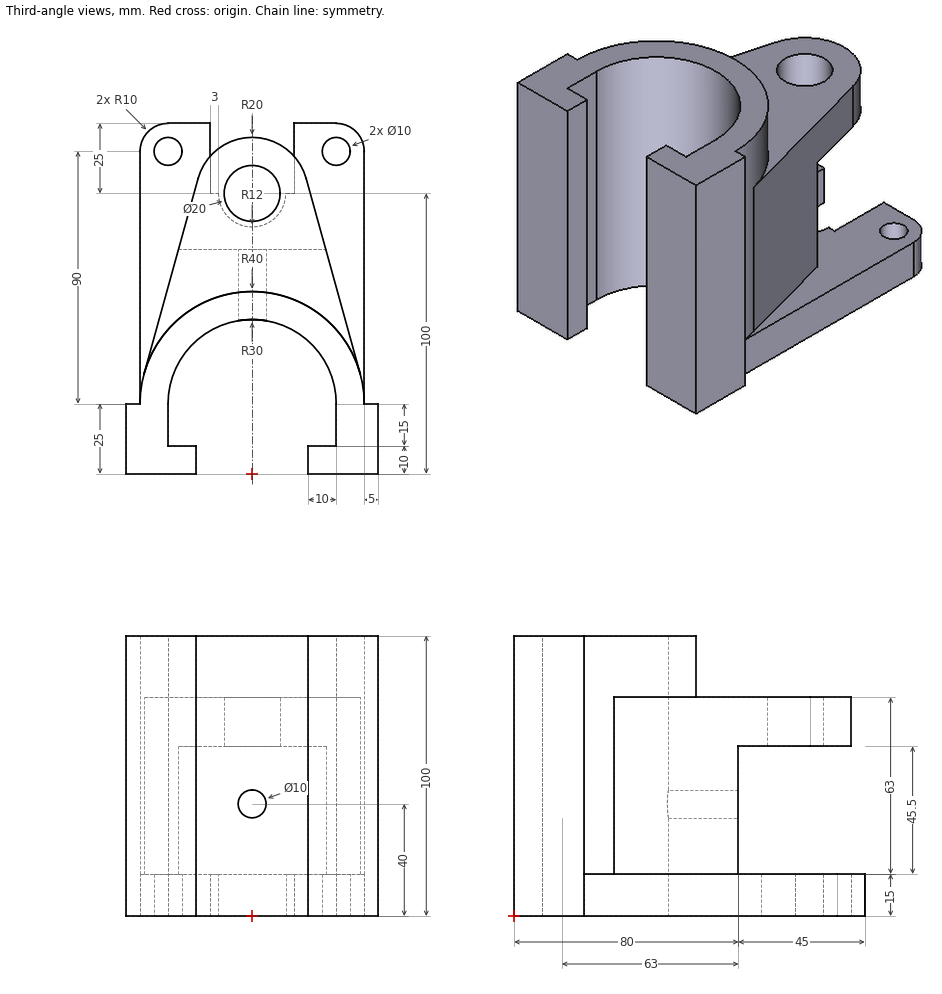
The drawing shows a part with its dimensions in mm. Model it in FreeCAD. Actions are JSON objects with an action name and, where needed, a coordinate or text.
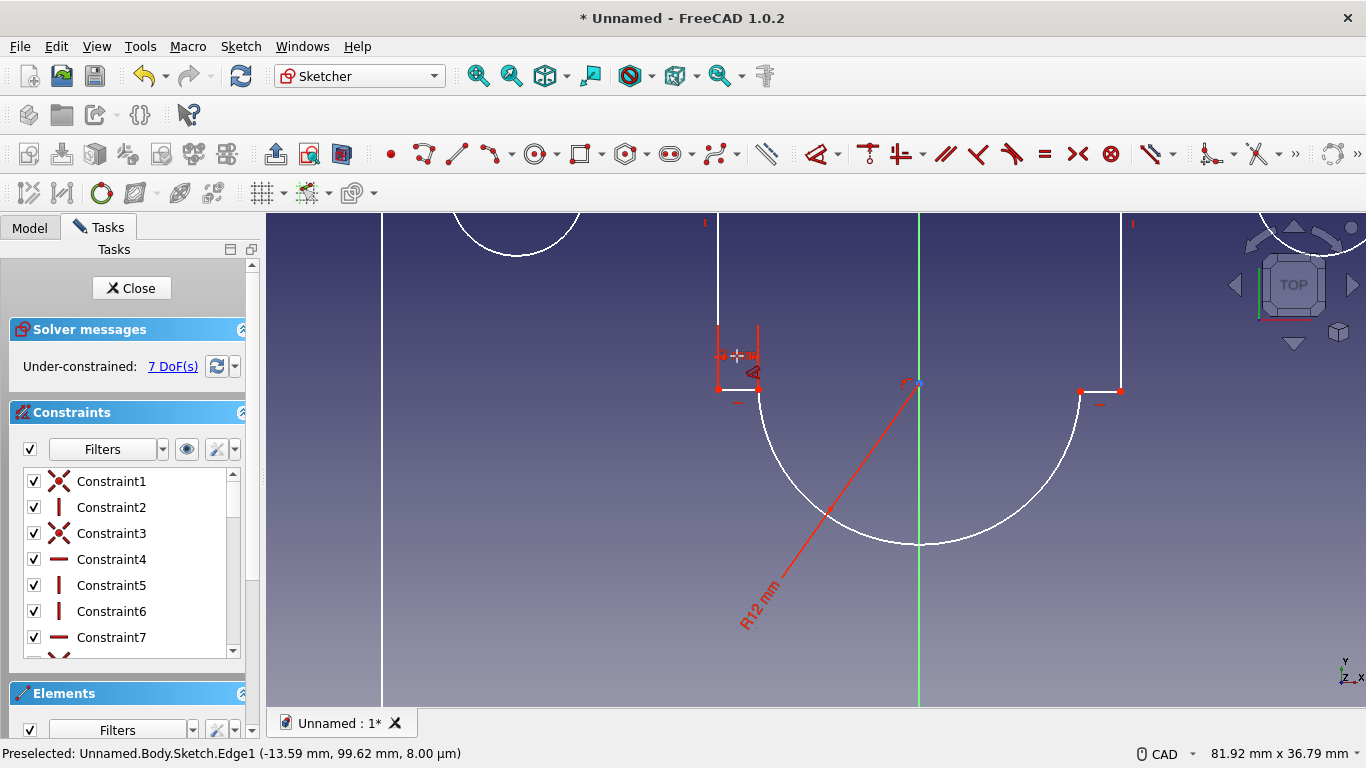
{"action": "scroll", "coordinate": [704, 352], "scroll_direction": "down", "scroll_amount": 8}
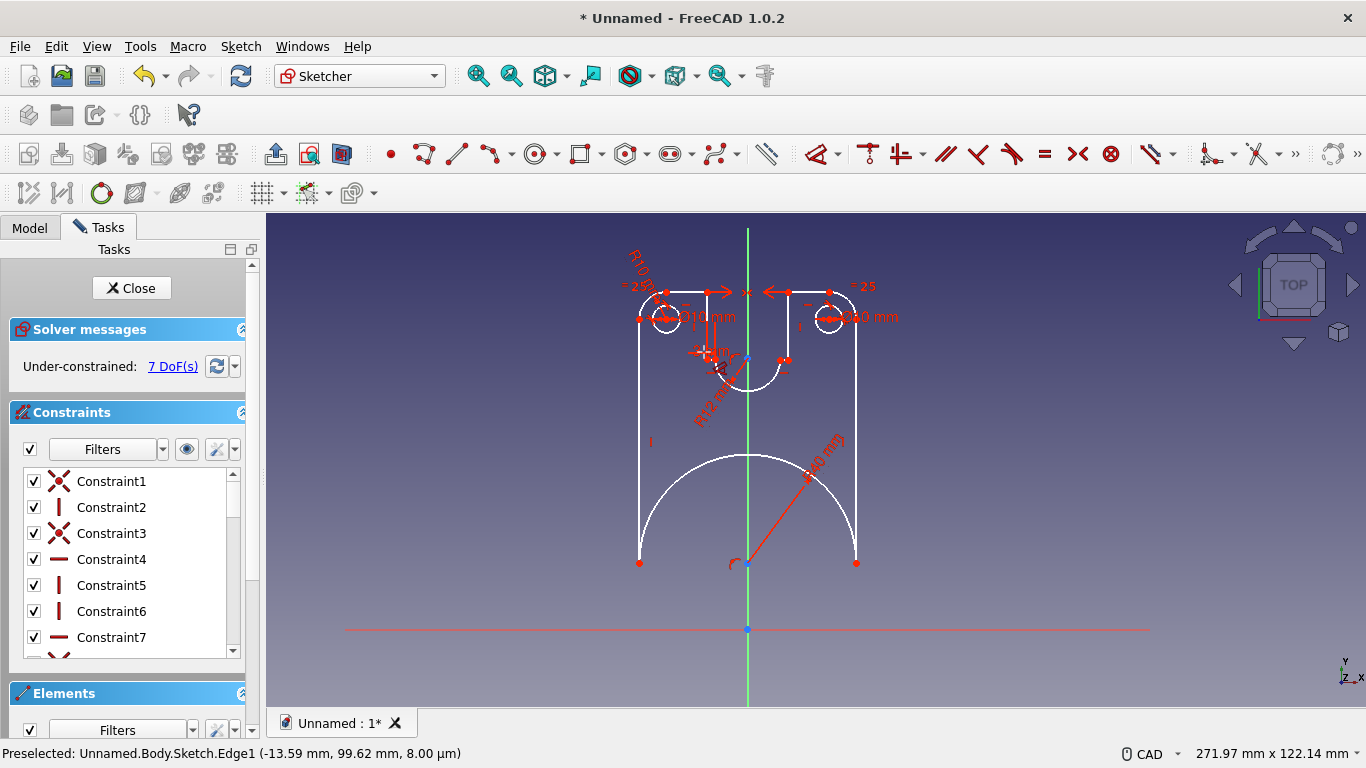
{"action": "left_click", "coordinate": [707, 340]}
{"action": "left_click", "coordinate": [765, 326]}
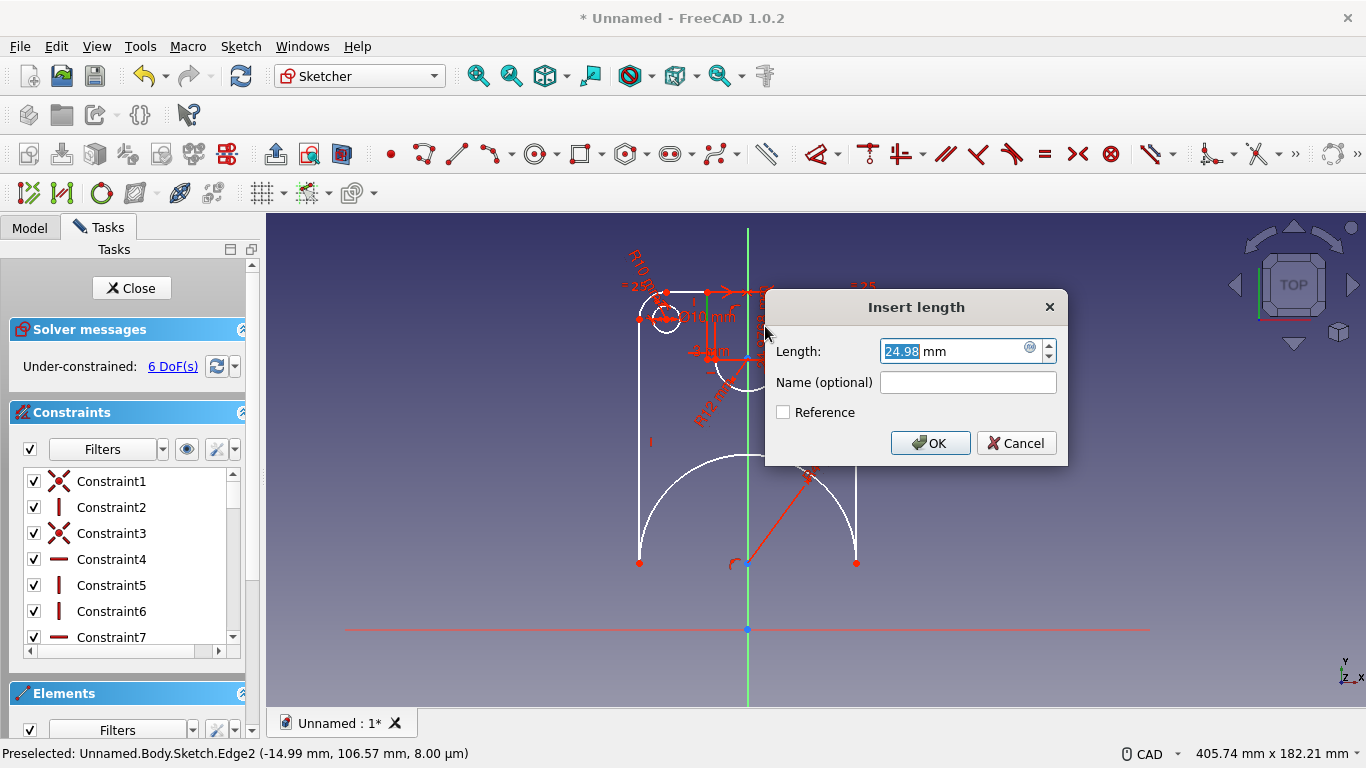
{"action": "type", "text": "25"}
{"action": "key", "text": "Return"}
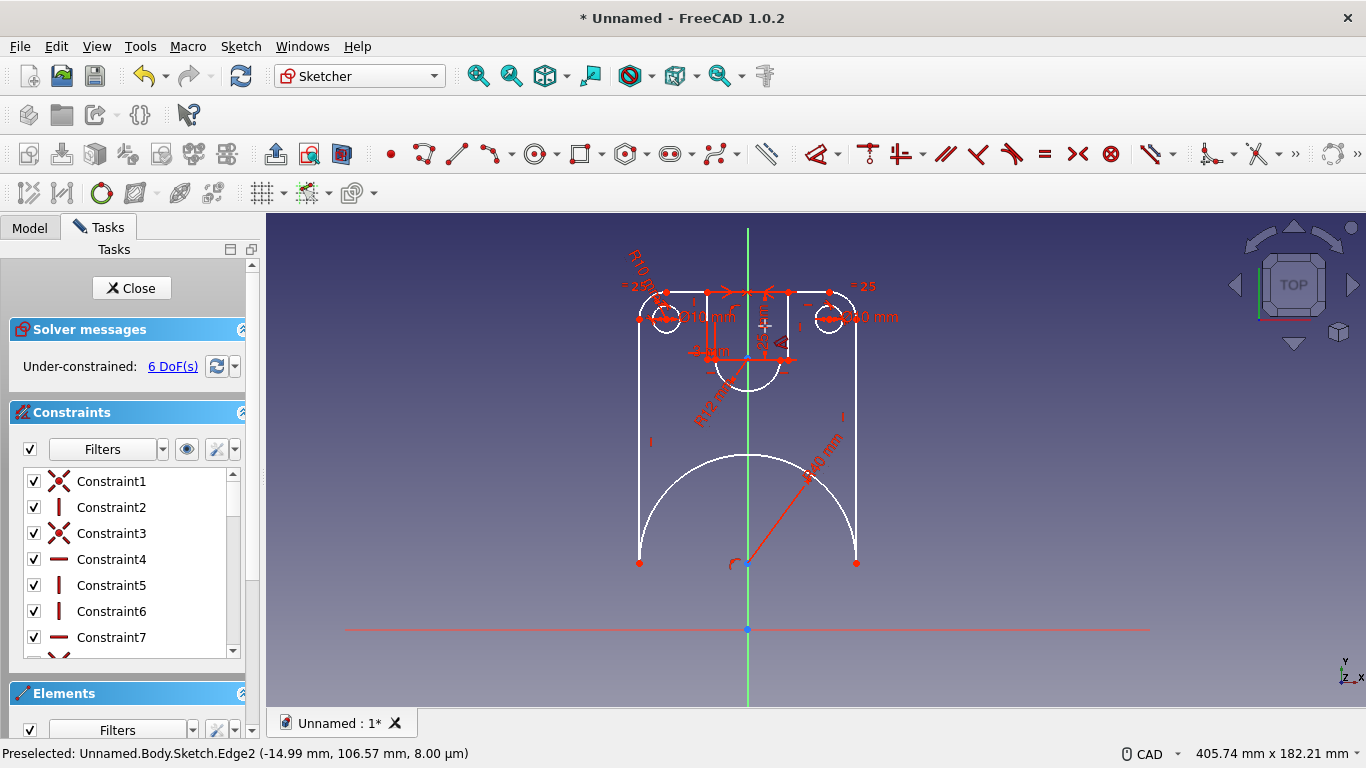
{"action": "left_click", "coordinate": [639, 392]}
{"action": "left_click", "coordinate": [605, 441]}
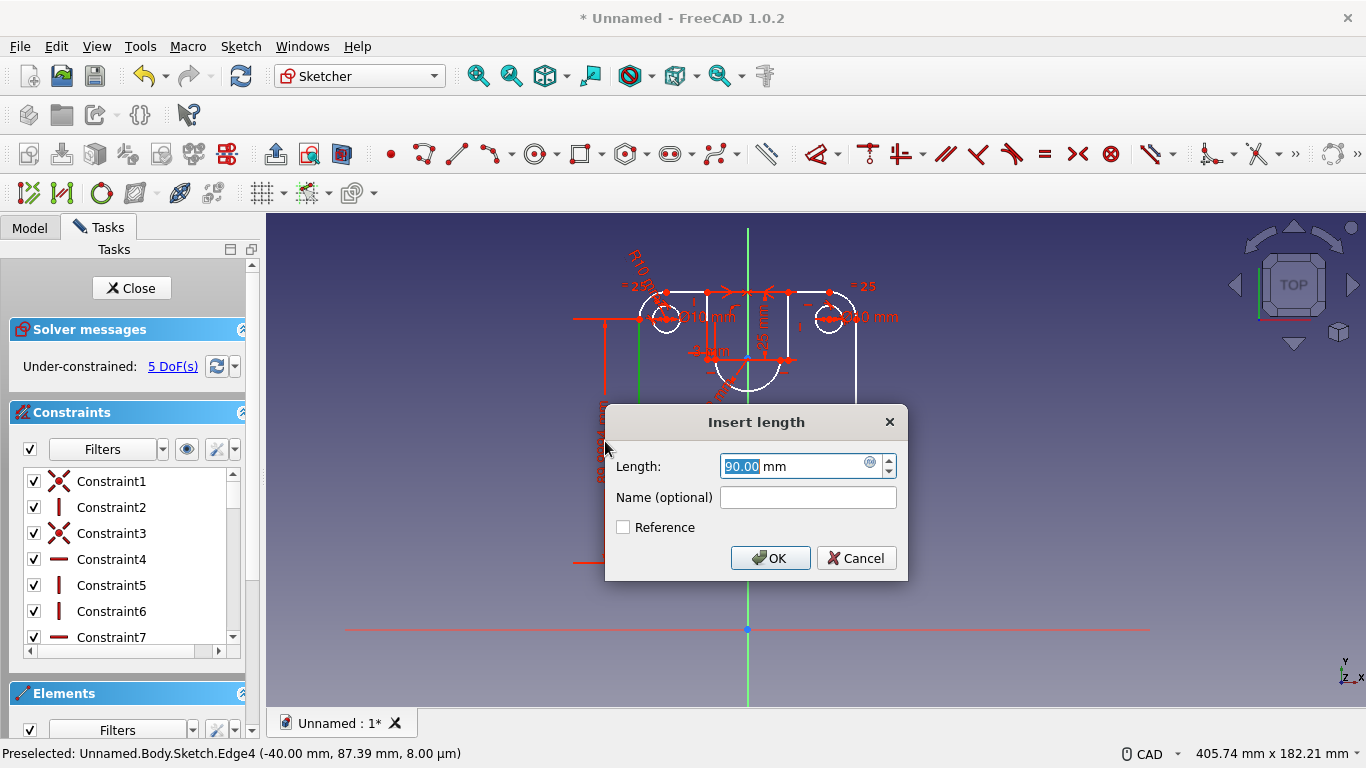
{"action": "type", "text": "90"}
{"action": "key", "text": "Return"}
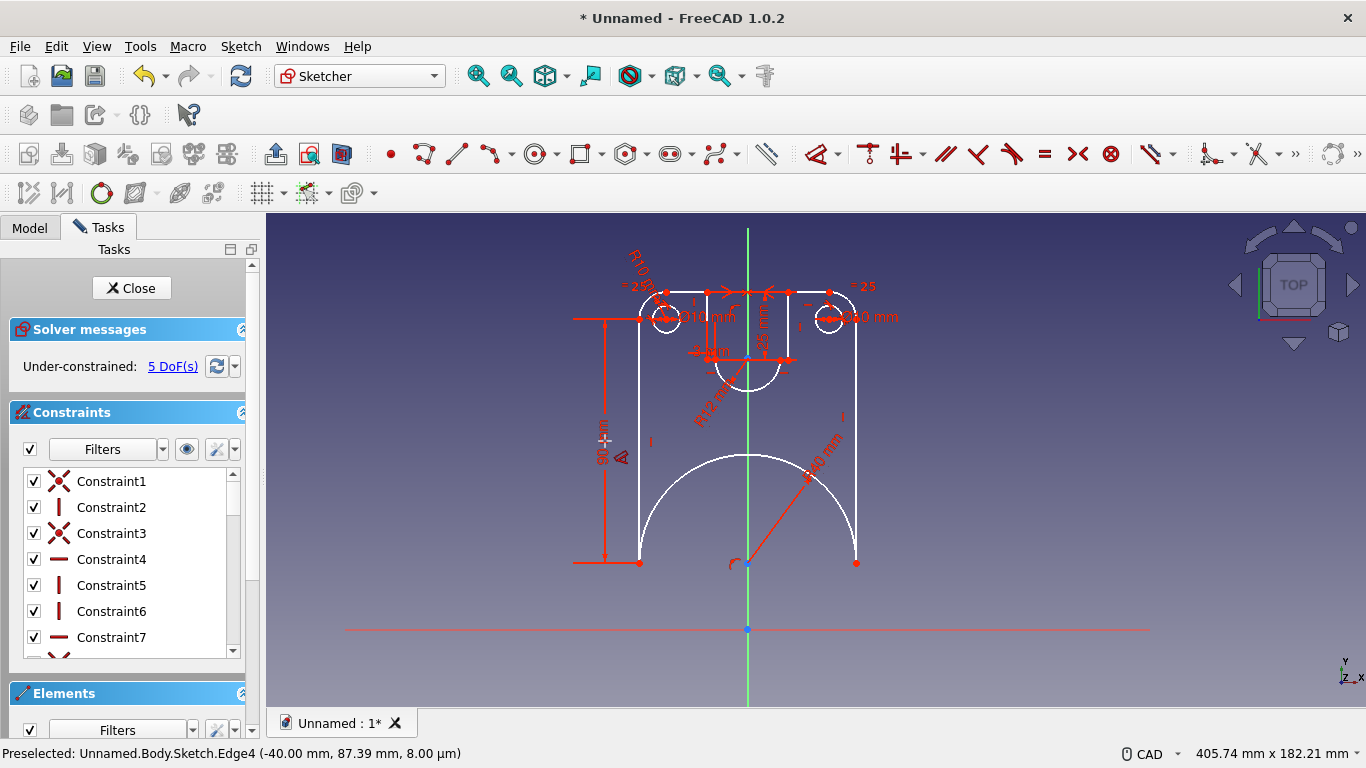
{"action": "left_click", "coordinate": [856, 490]}
{"action": "left_click", "coordinate": [890, 385]}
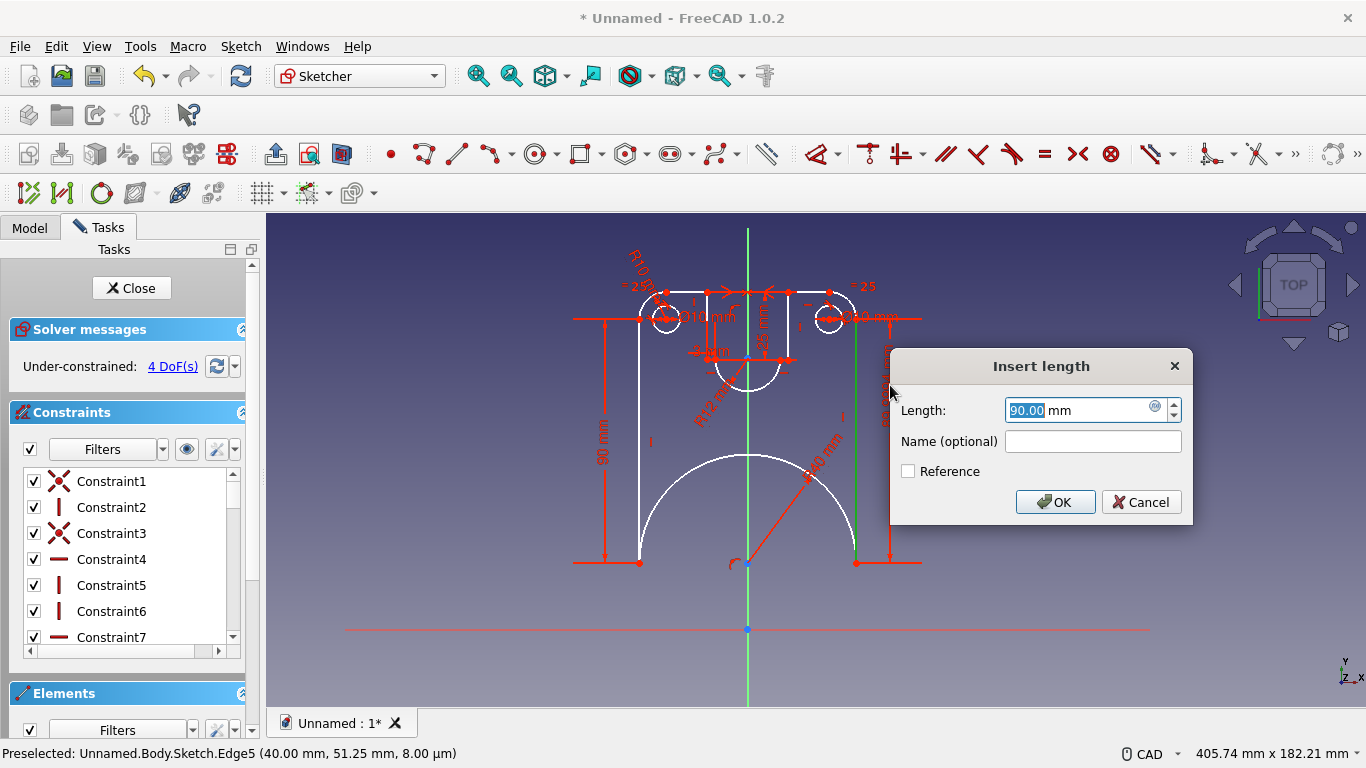
{"action": "type", "text": "90"}
{"action": "key", "text": "Return"}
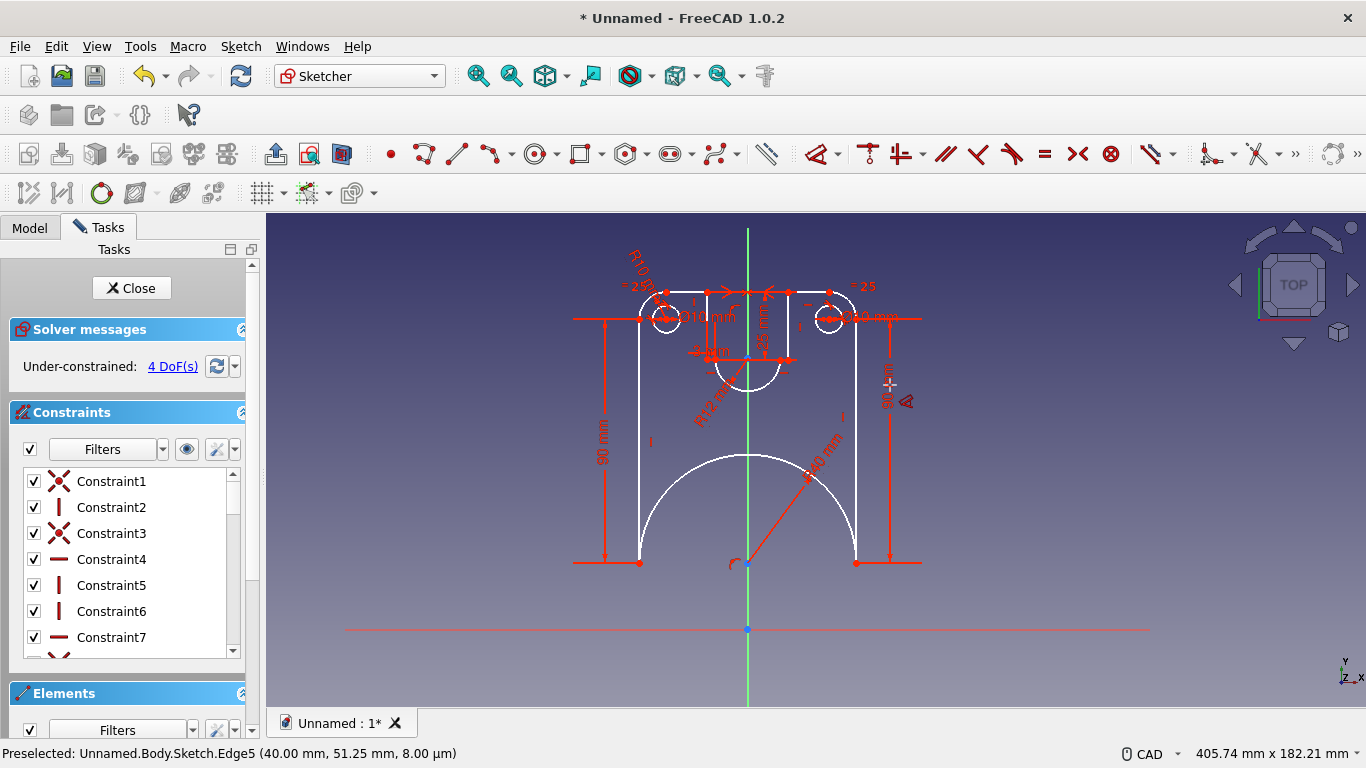
{"action": "left_click", "coordinate": [788, 313]}
{"action": "left_click", "coordinate": [822, 350]}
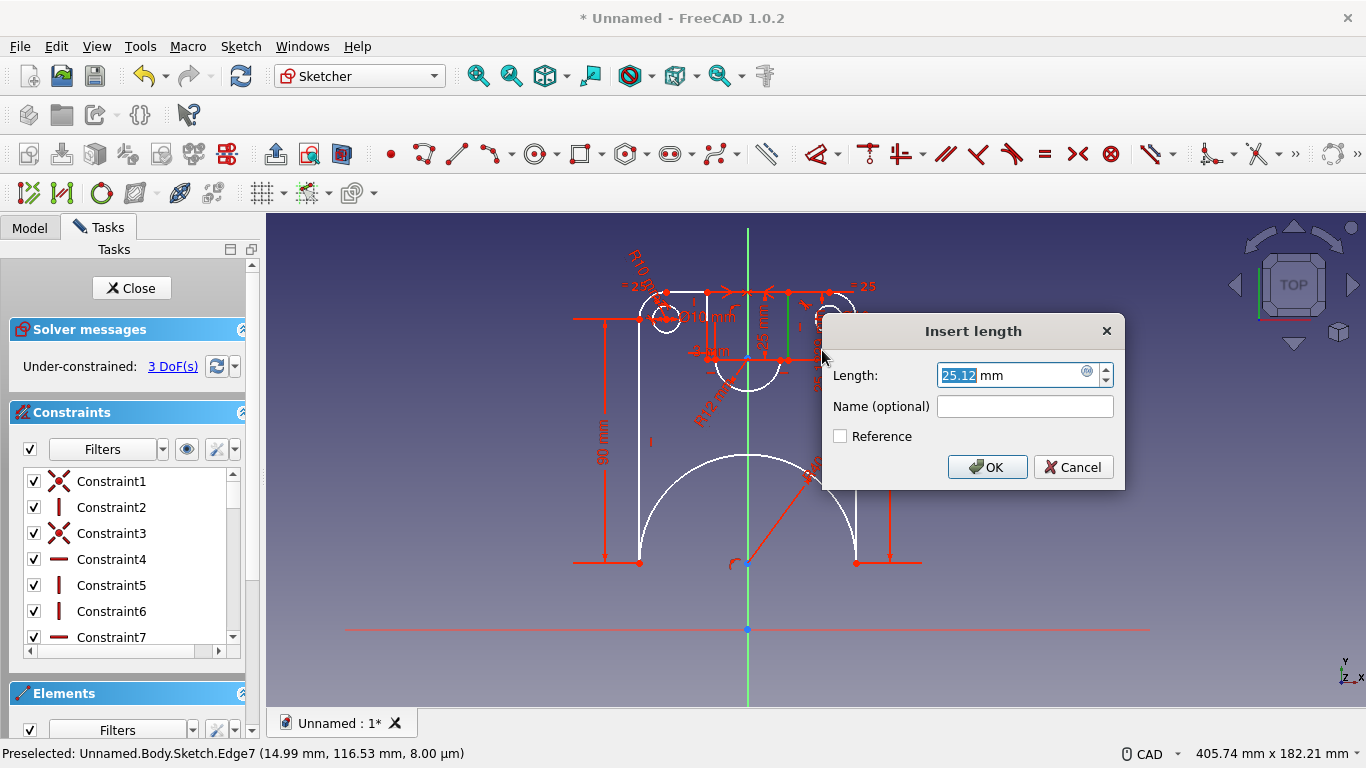
{"action": "type", "text": "25"}
{"action": "key", "text": "Return"}